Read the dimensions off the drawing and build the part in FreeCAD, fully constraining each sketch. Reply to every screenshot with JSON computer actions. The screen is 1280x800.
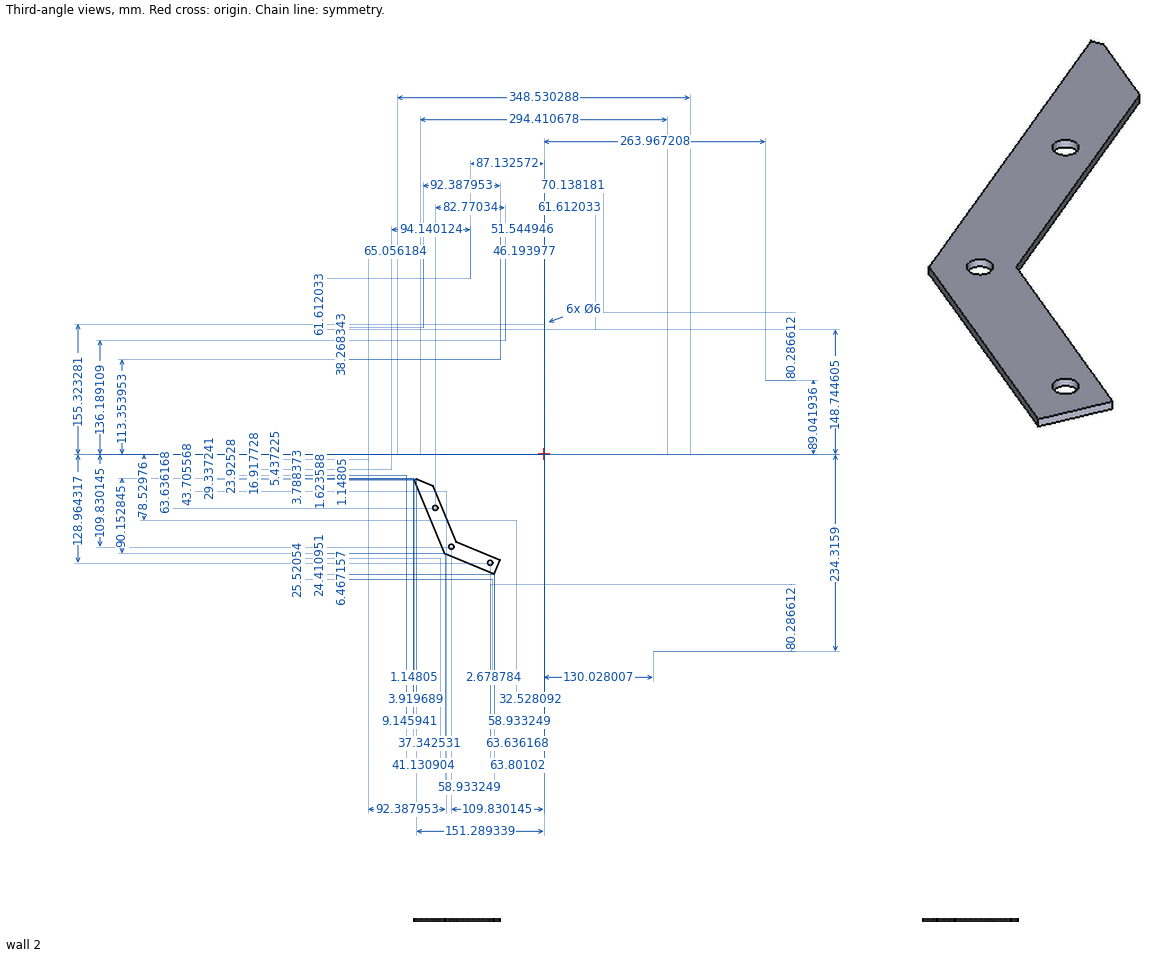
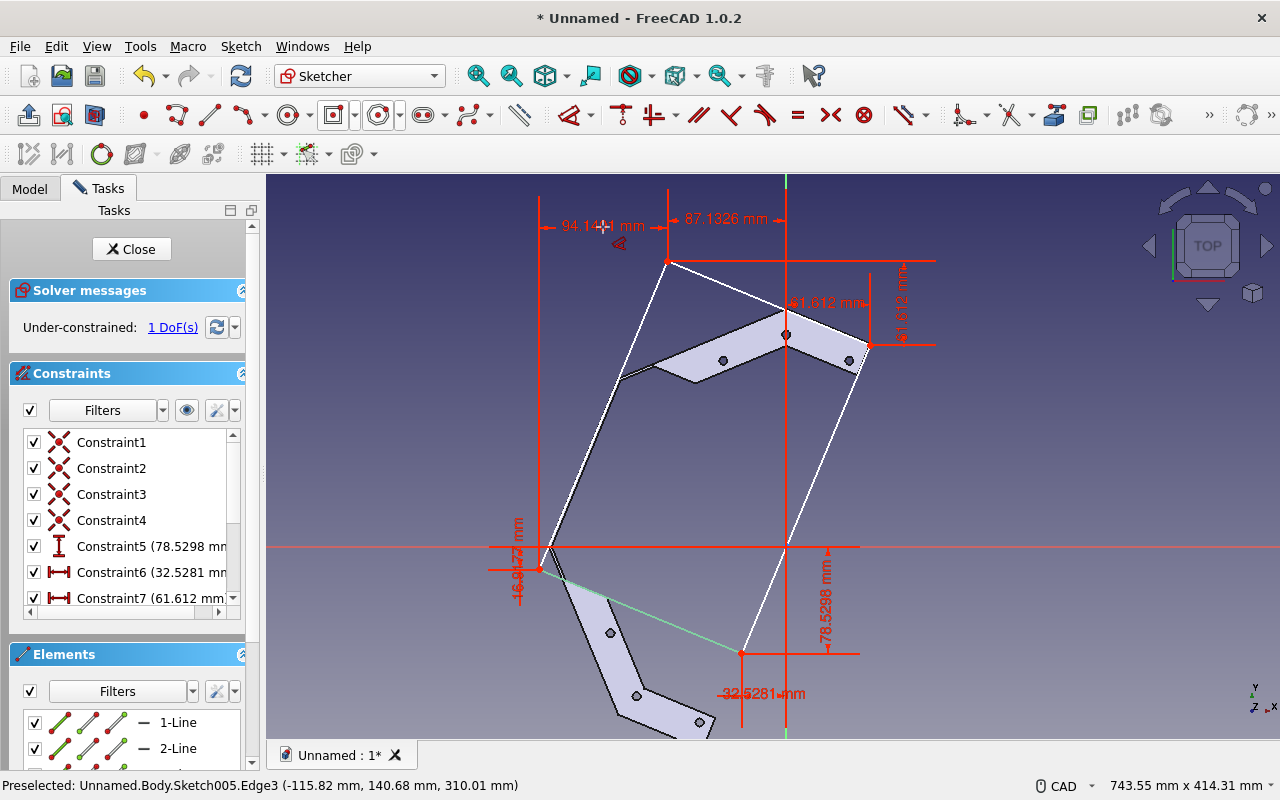
{"action": "left_click", "coordinate": [870, 345]}
{"action": "left_click", "coordinate": [904, 446]}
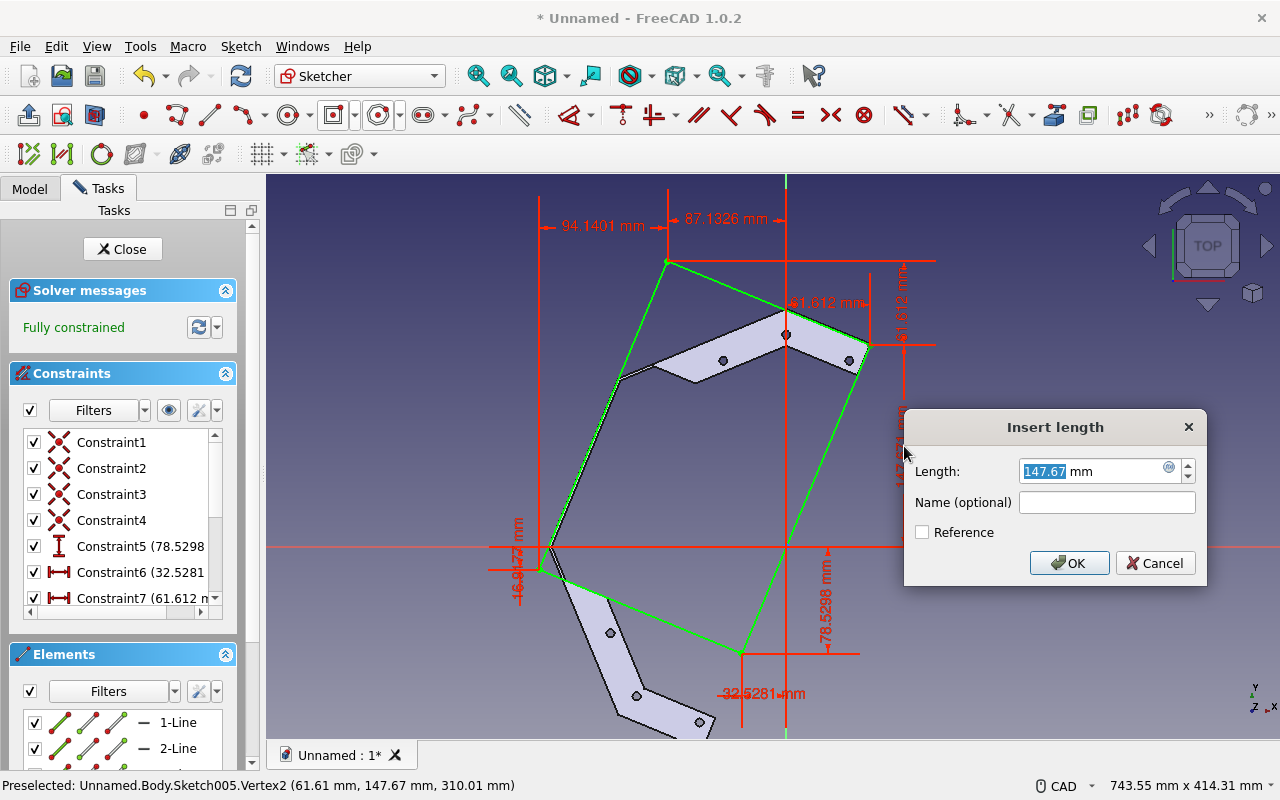
{"action": "type", "text": "148.744605"}
{"action": "key", "text": "Return"}
{"action": "key", "text": "Escape"}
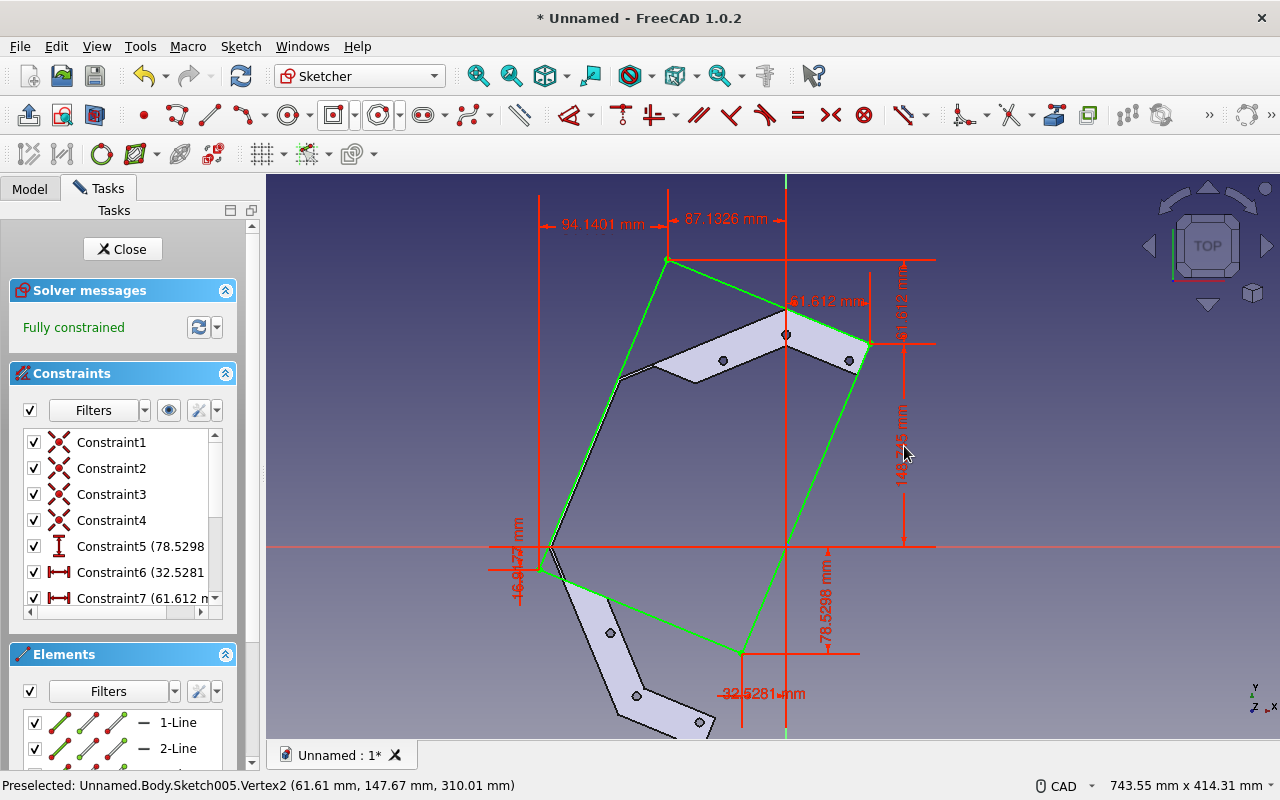
{"action": "left_click", "coordinate": [123, 249]}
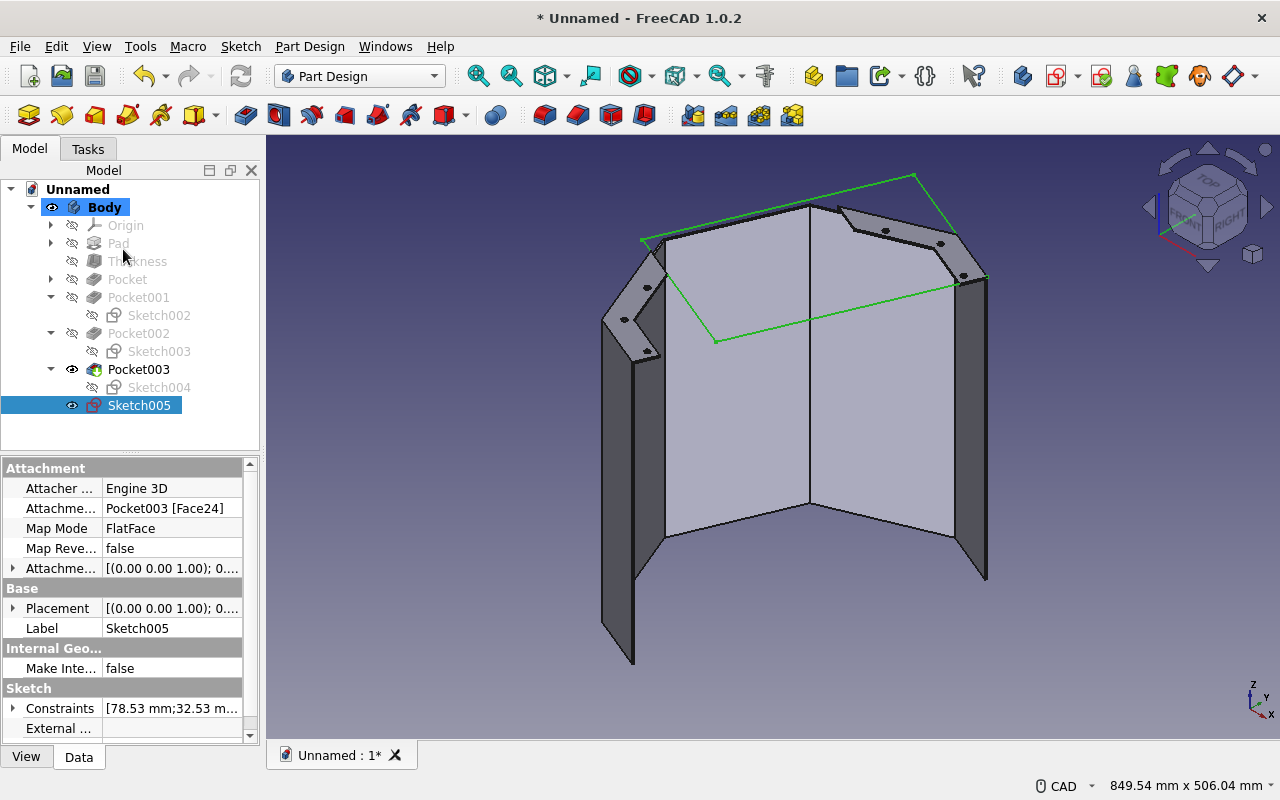
{"action": "left_click", "coordinate": [246, 116]}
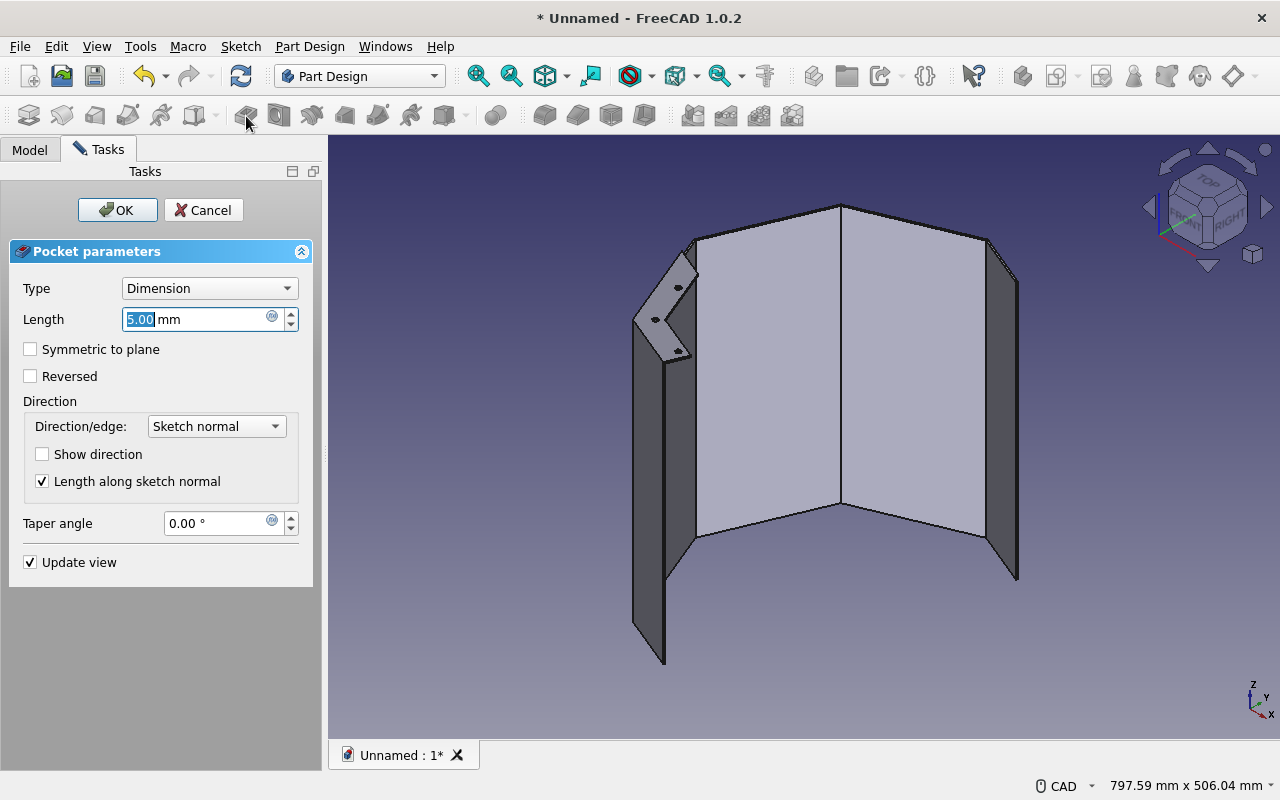
{"action": "left_click", "coordinate": [210, 288]}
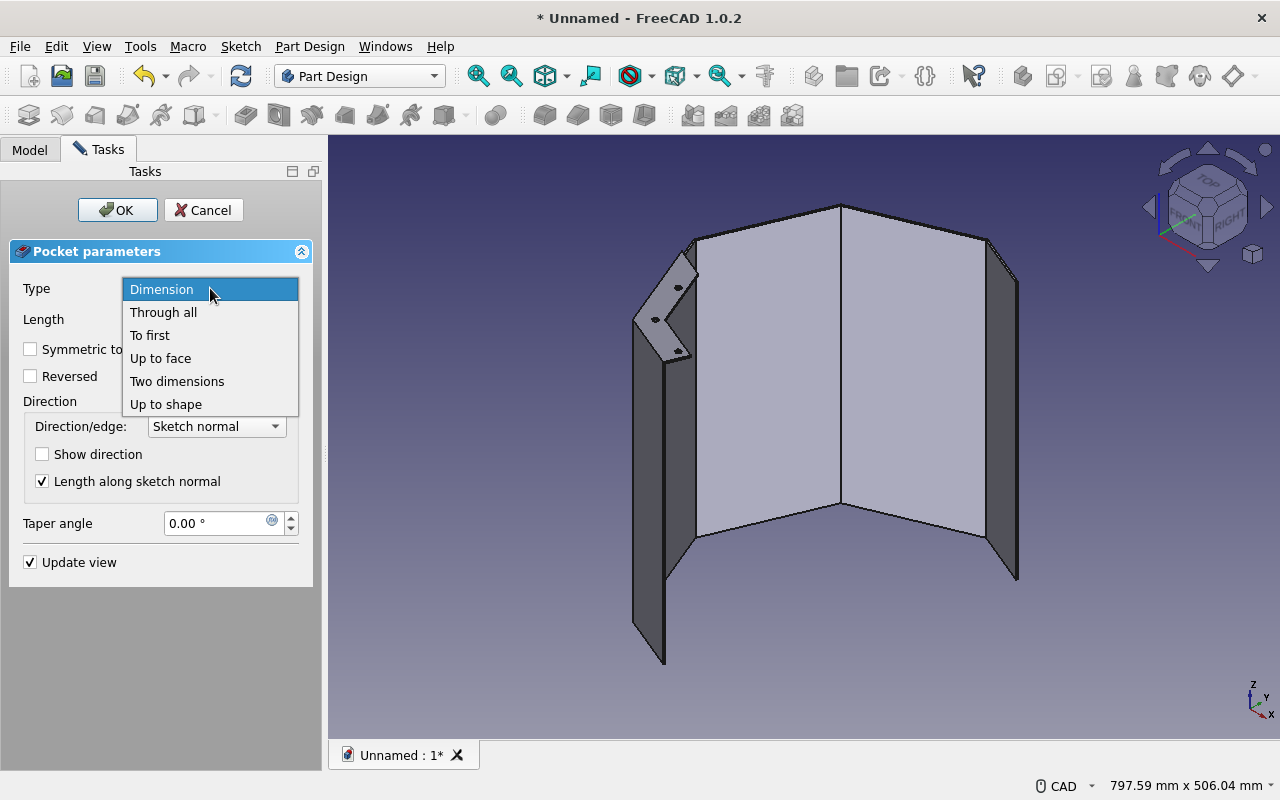
{"action": "left_click", "coordinate": [208, 312]}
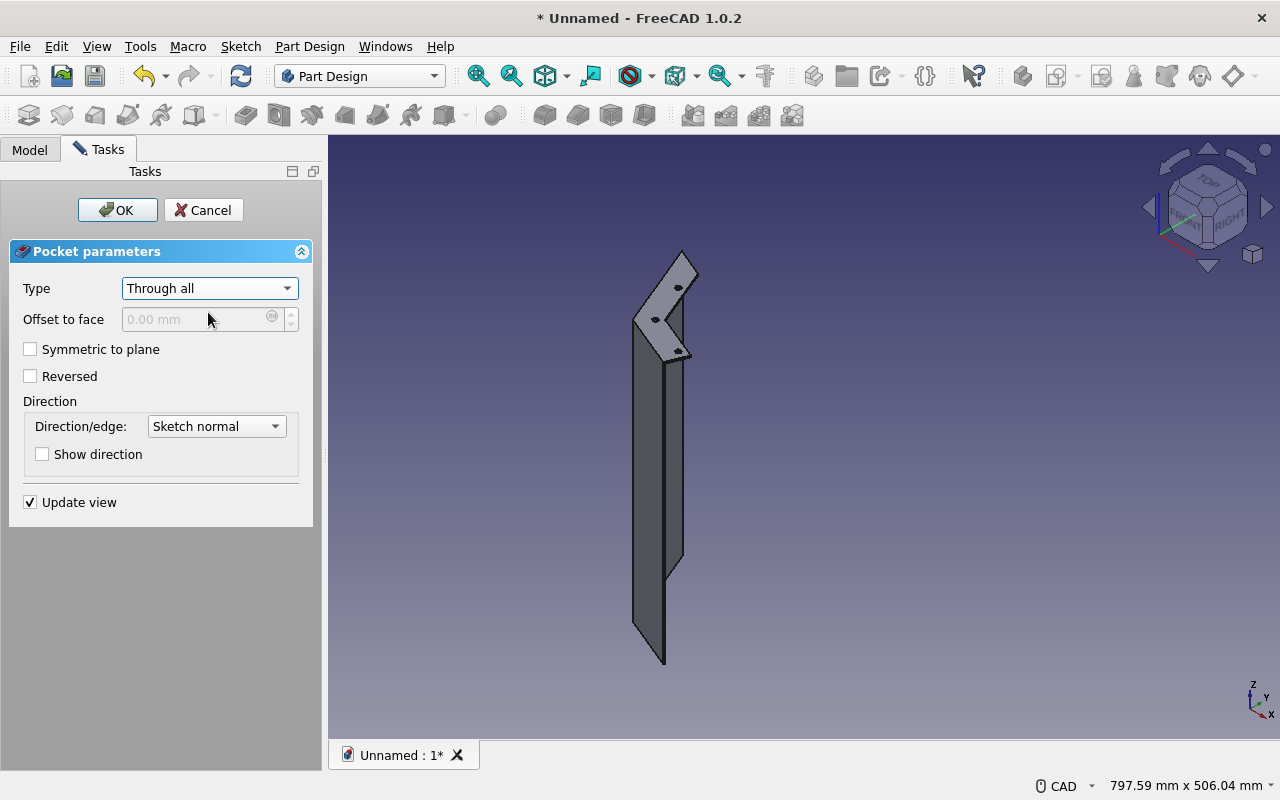
{"action": "left_click", "coordinate": [118, 210]}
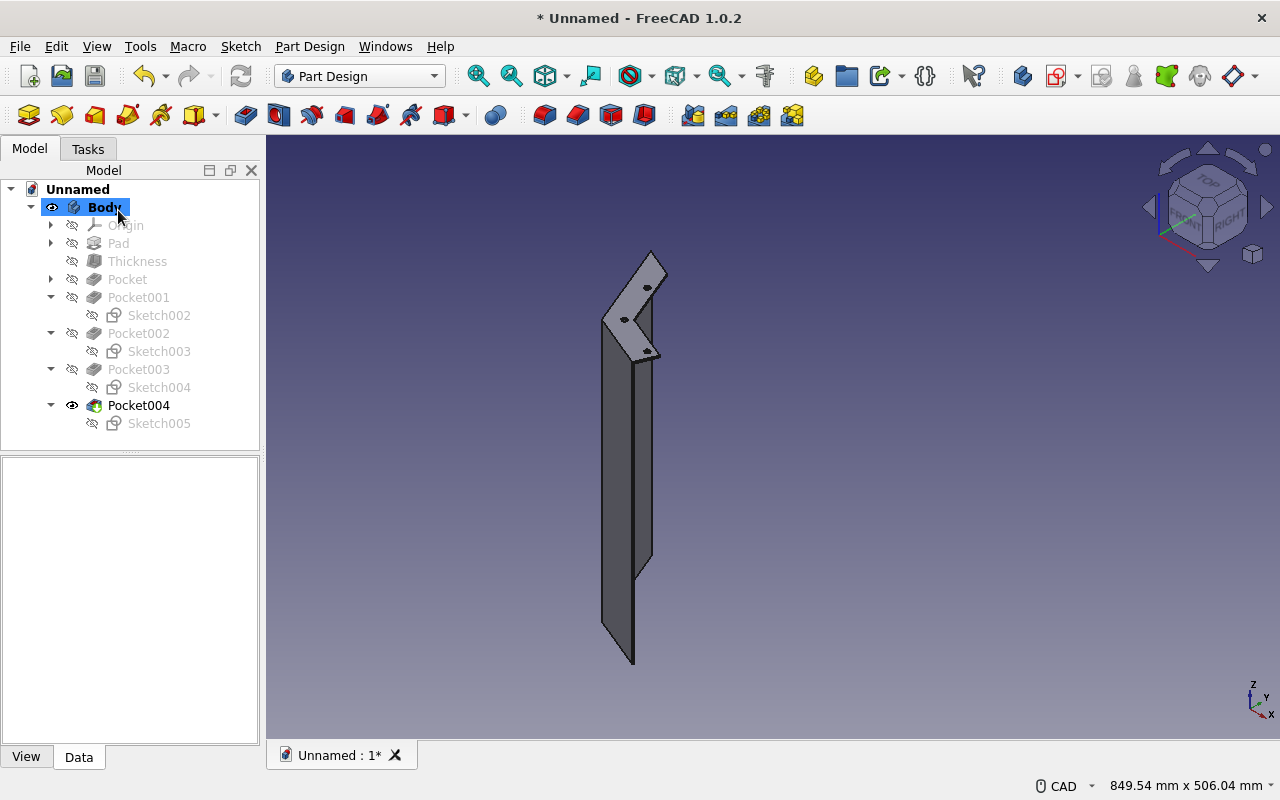
{"action": "left_click", "coordinate": [649, 275]}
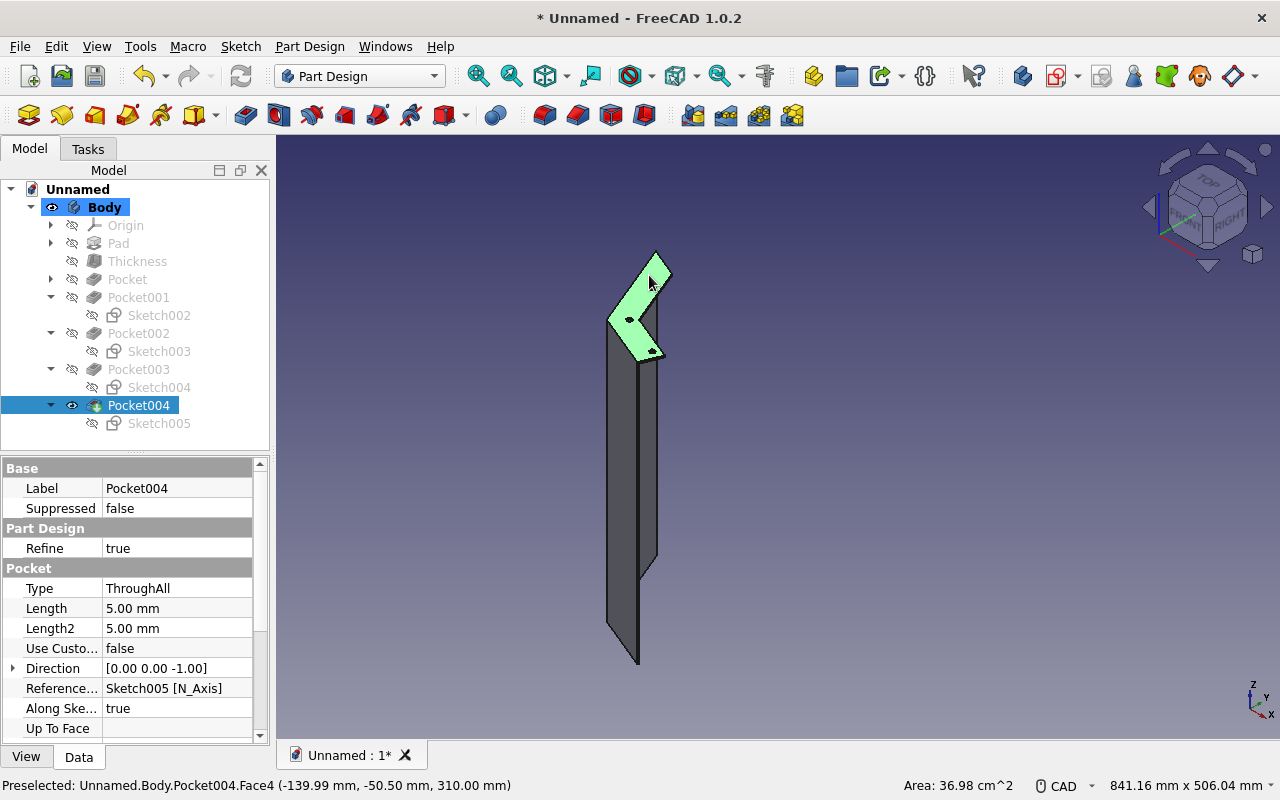
{"action": "left_click", "coordinate": [1056, 76]}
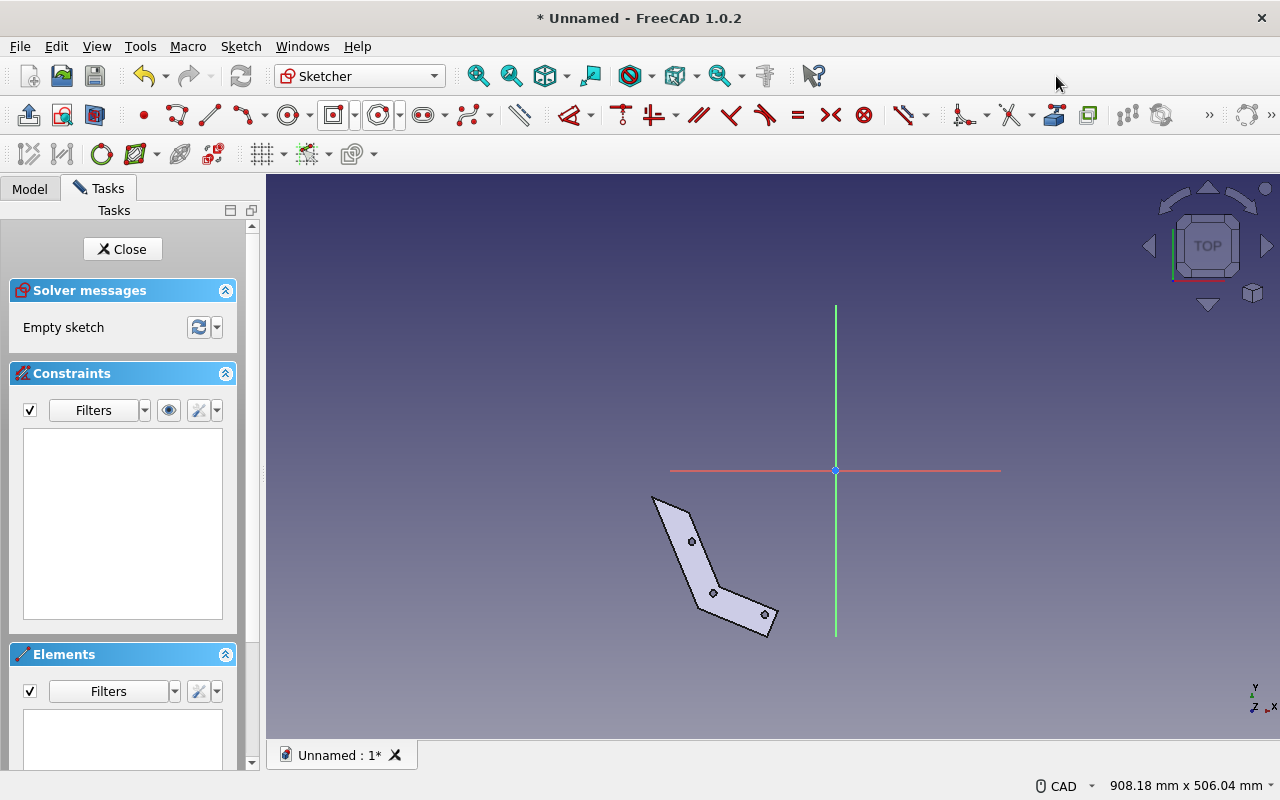
{"action": "scroll", "coordinate": [776, 633], "scroll_direction": "up", "scroll_amount": 4}